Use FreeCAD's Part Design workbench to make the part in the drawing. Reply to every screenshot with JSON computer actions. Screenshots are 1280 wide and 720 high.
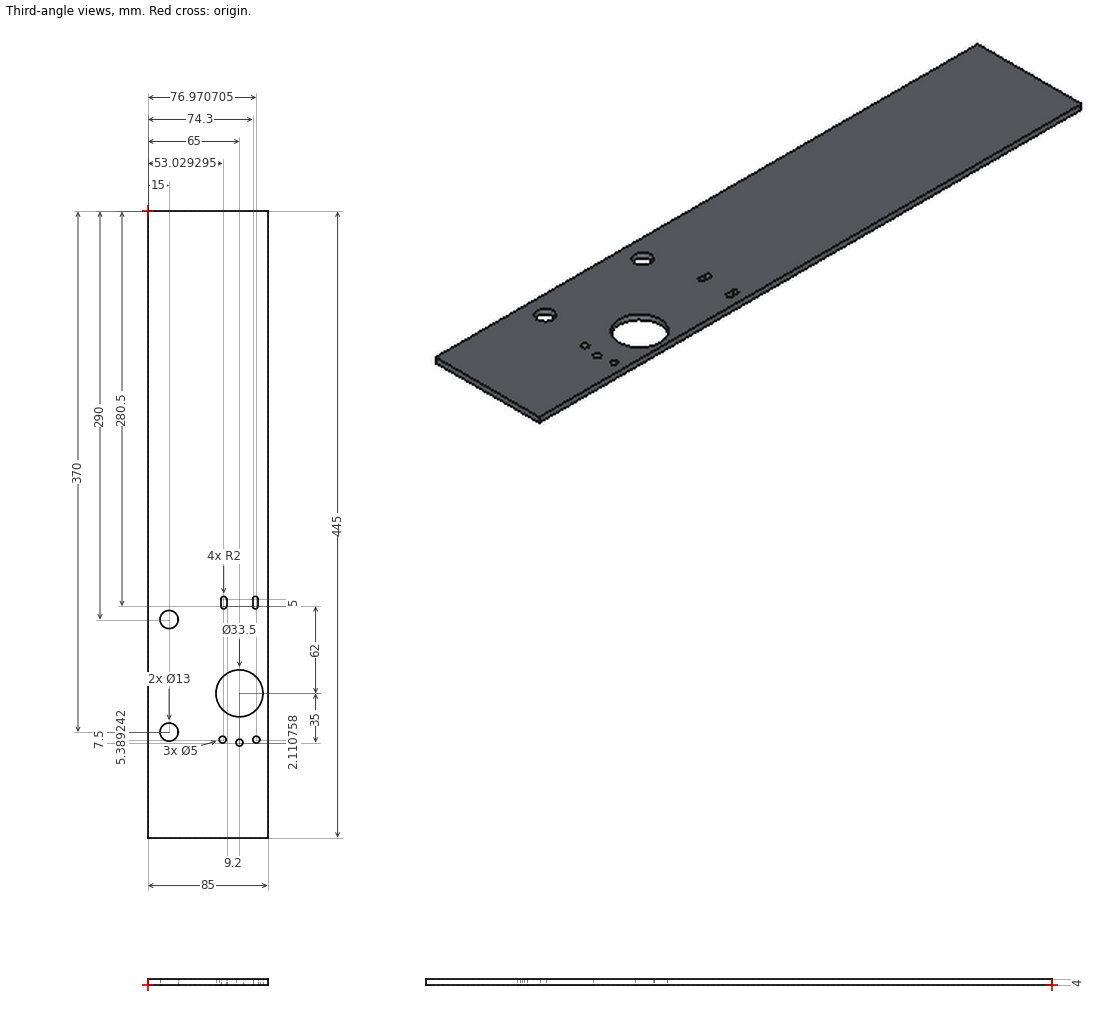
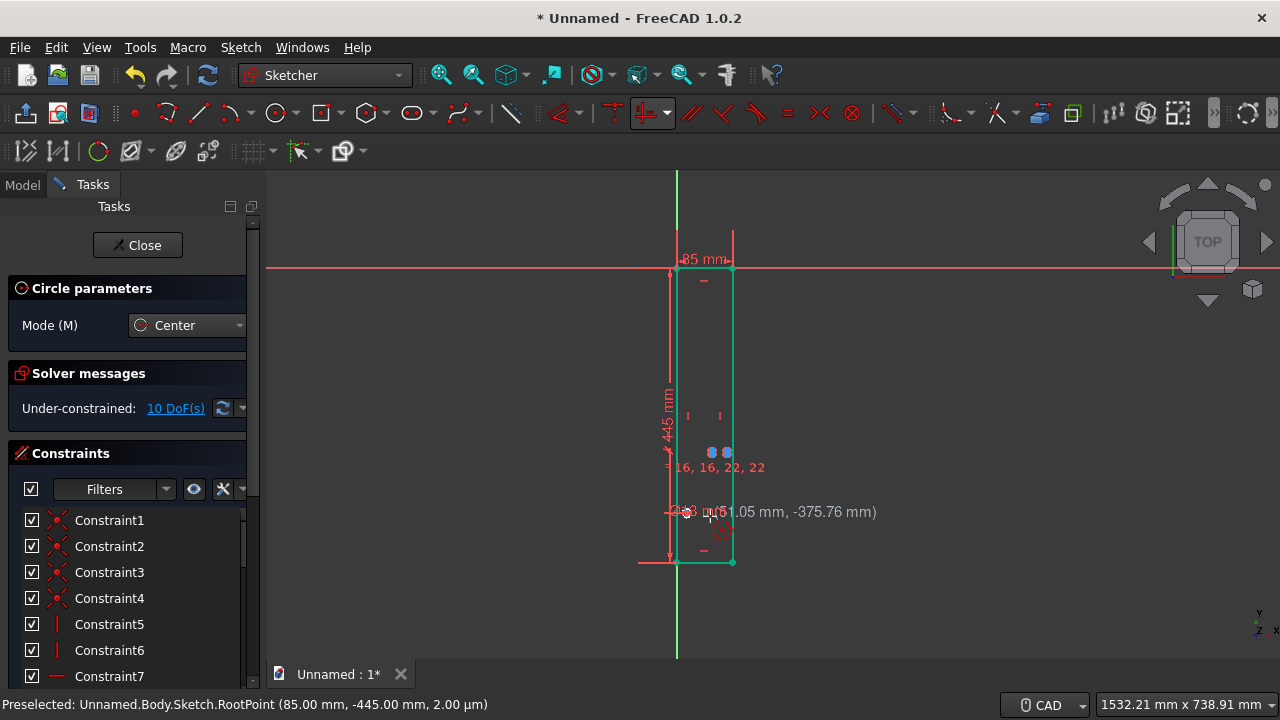
{"action": "left_click", "coordinate": [712, 516]}
{"action": "mouse_move", "coordinate": [713, 515]}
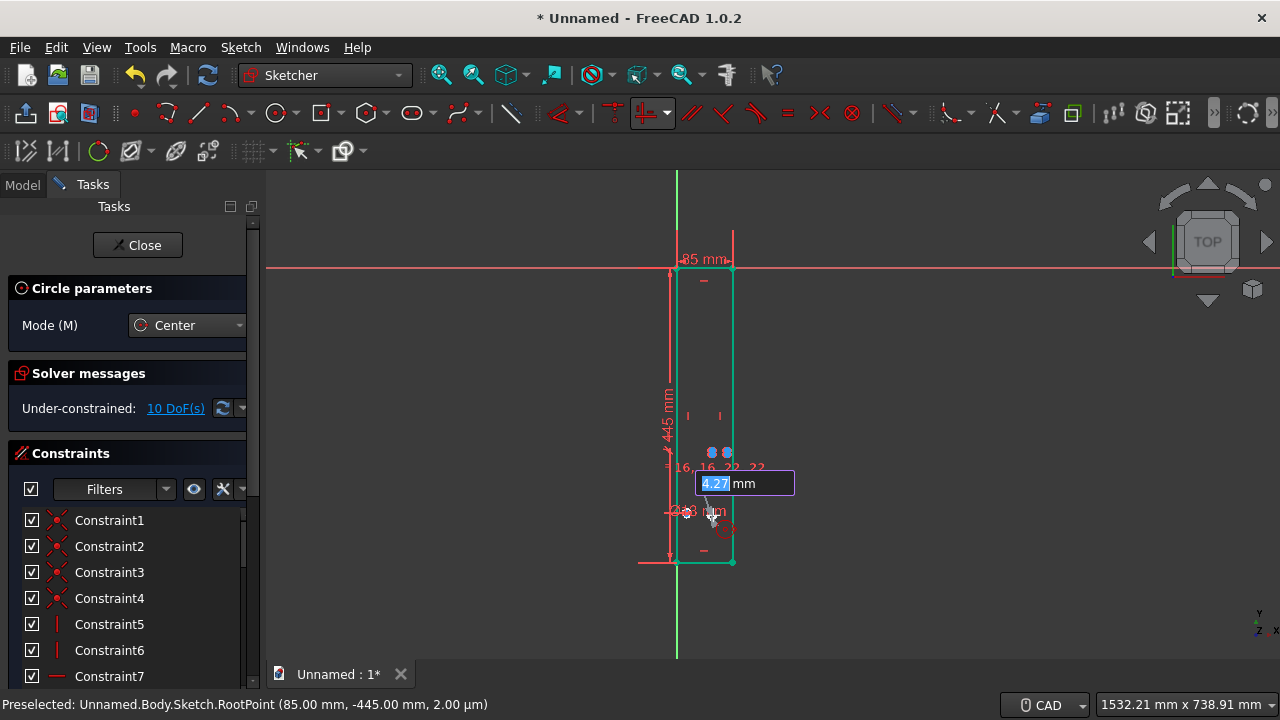
{"action": "type", "text": "5"}
{"action": "key", "text": "Return"}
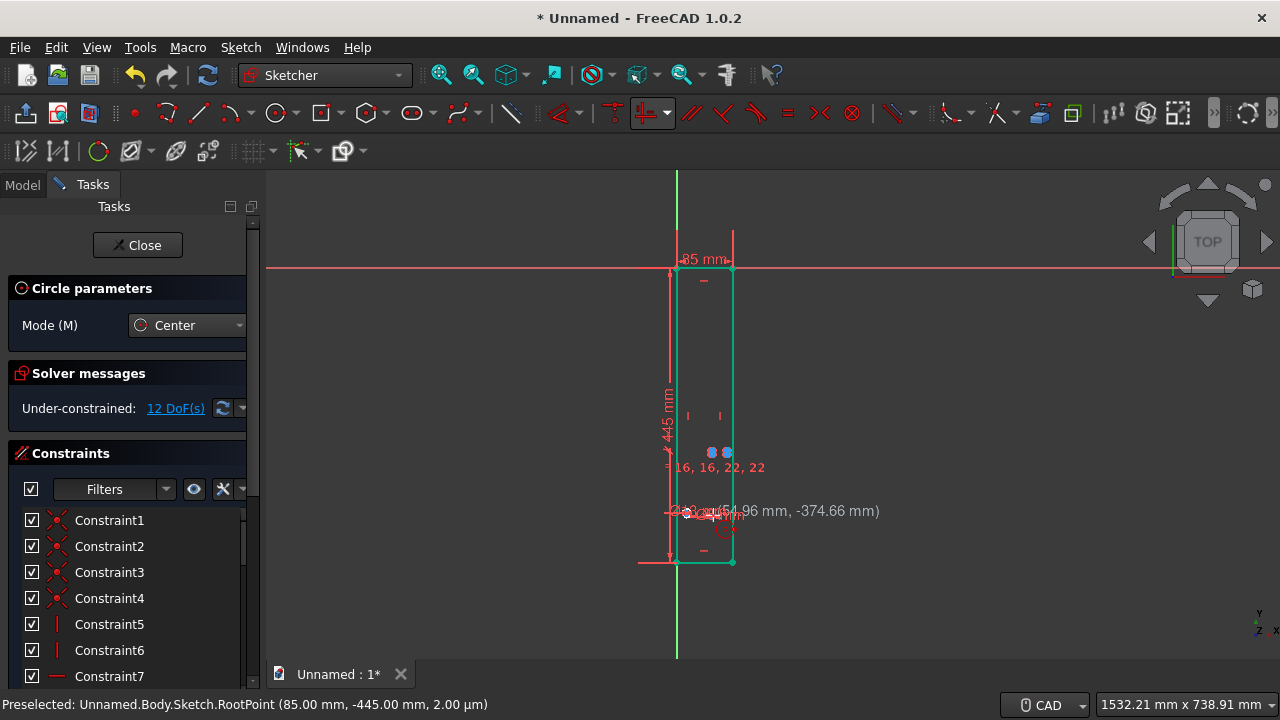
{"action": "scroll", "coordinate": [720, 518], "scroll_direction": "up", "scroll_amount": 14}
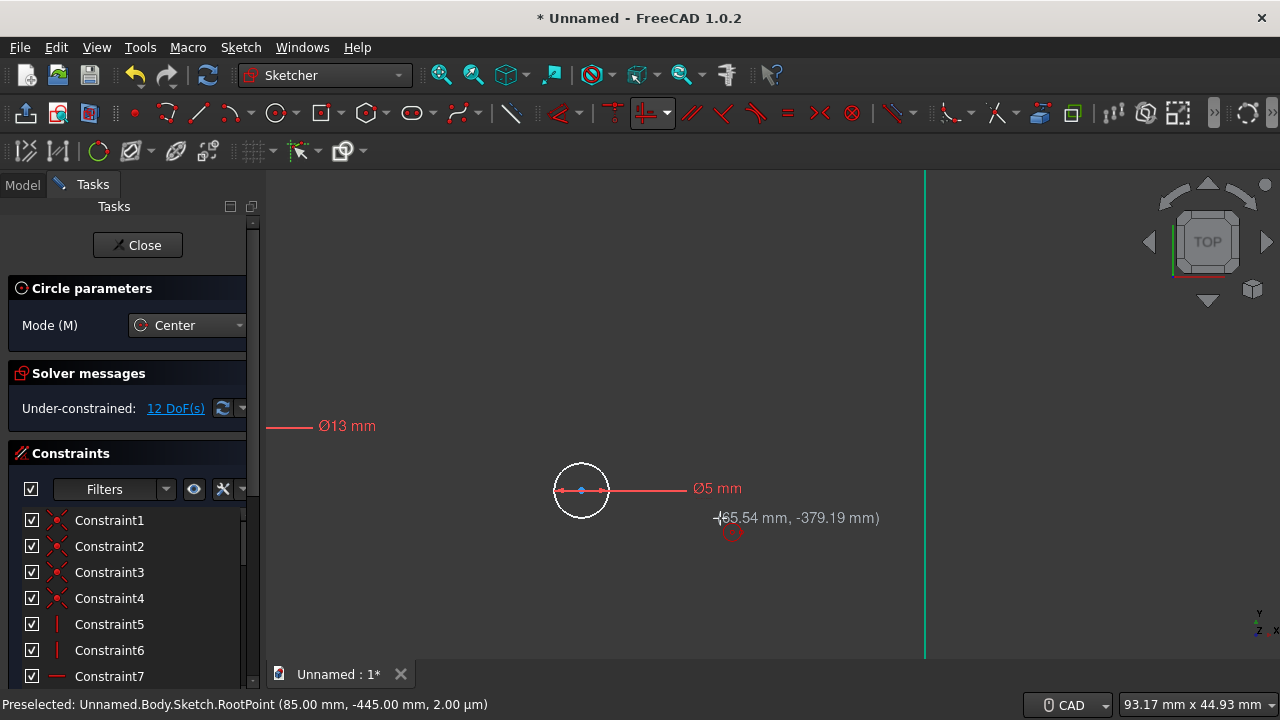
{"action": "scroll", "coordinate": [720, 518], "scroll_direction": "down", "scroll_amount": 14}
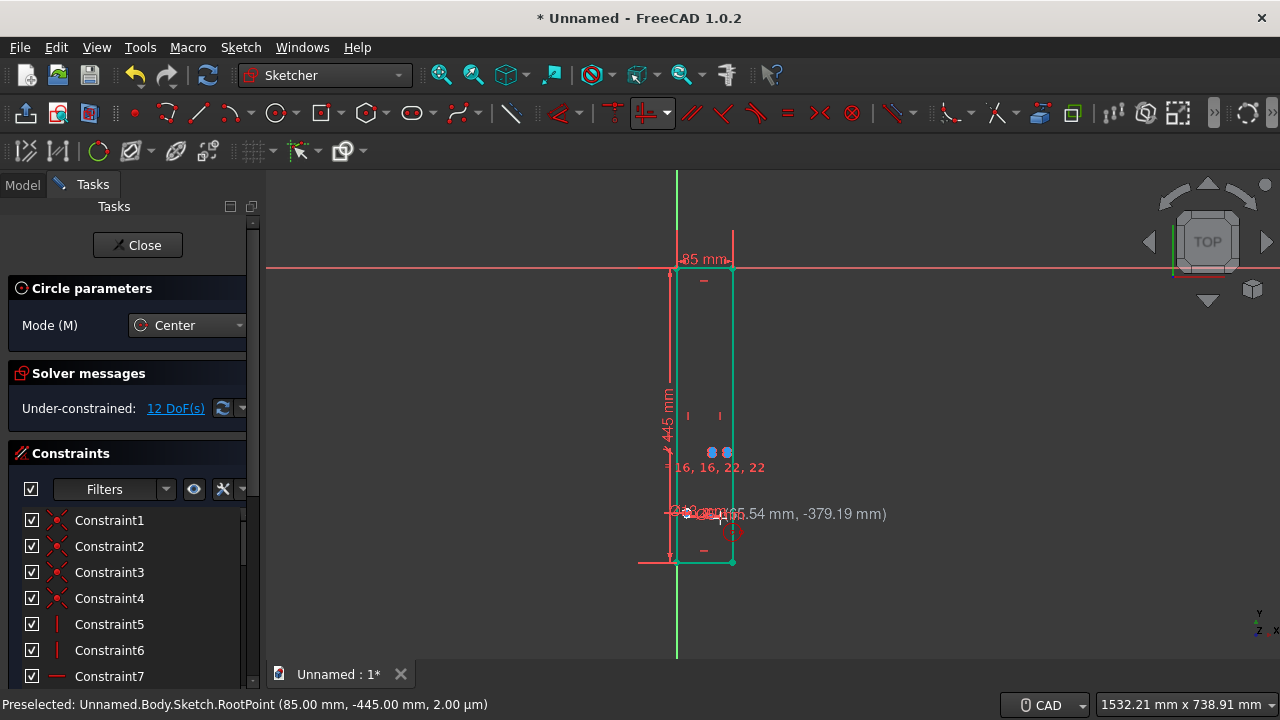
{"action": "scroll", "coordinate": [720, 518], "scroll_direction": "up", "scroll_amount": 5}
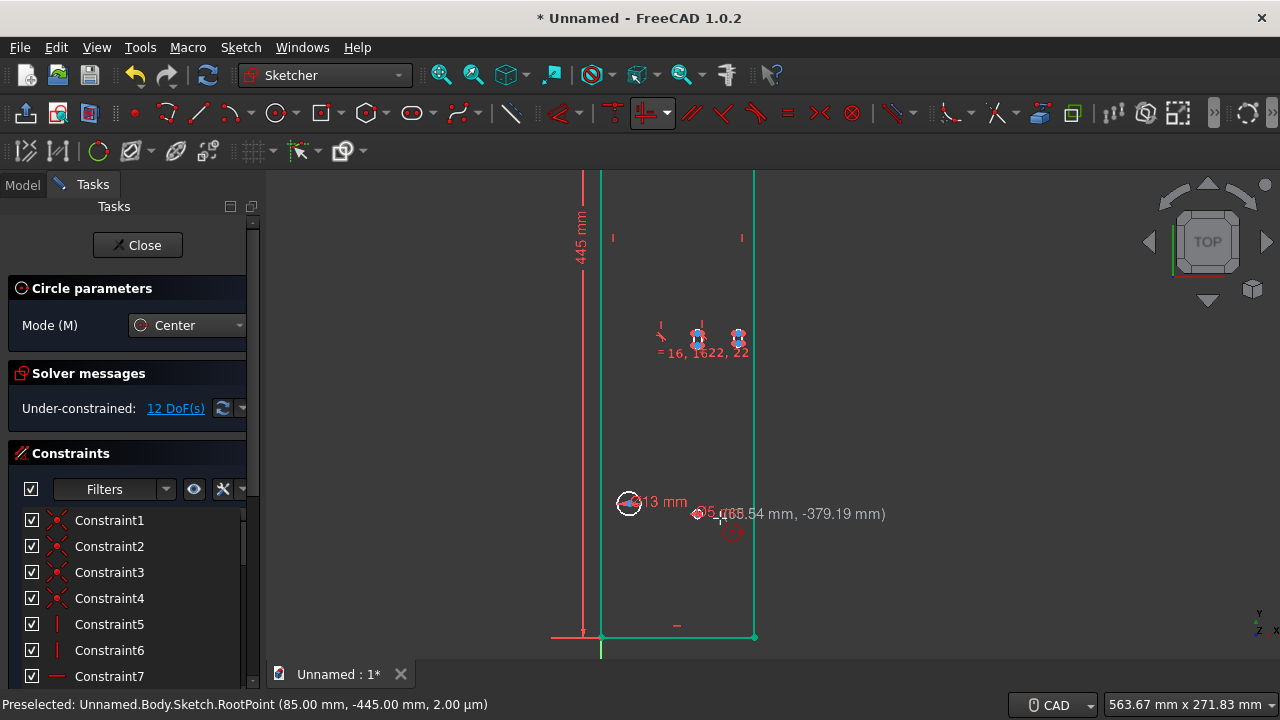
{"action": "left_click", "coordinate": [718, 516]}
{"action": "mouse_move", "coordinate": [721, 513]}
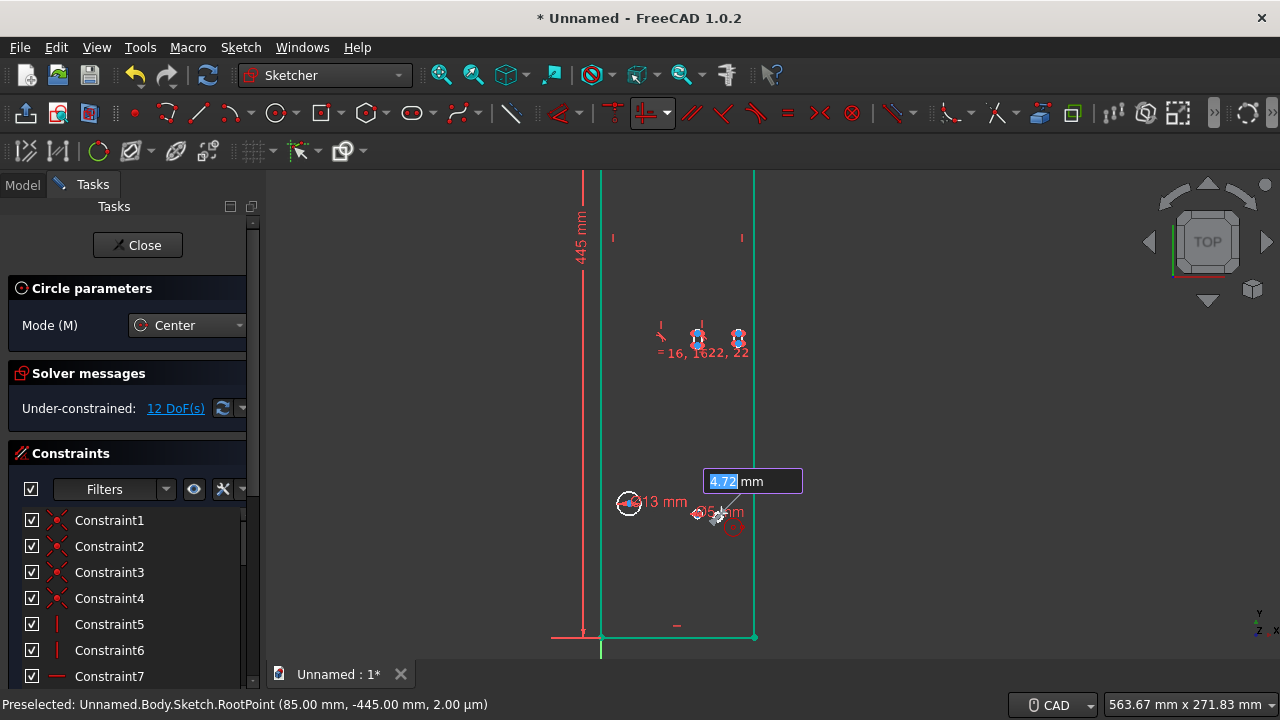
{"action": "type", "text": "5"}
{"action": "key", "text": "Return"}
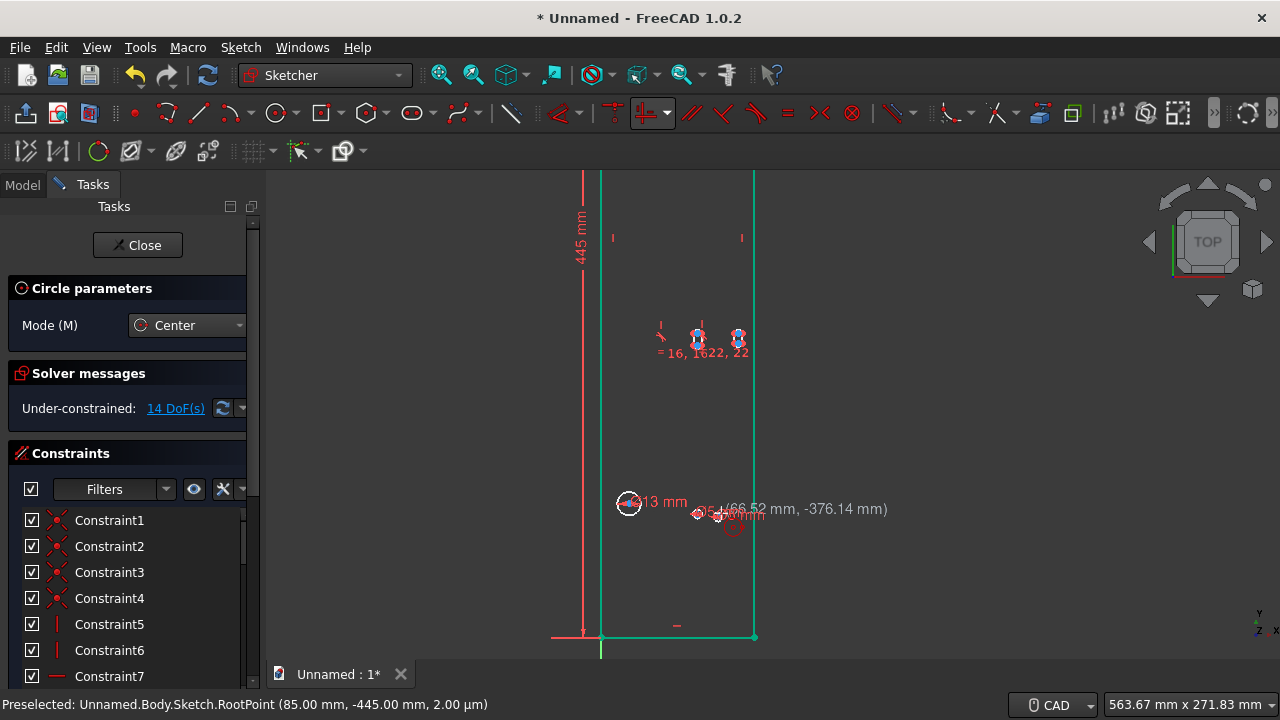
{"action": "scroll", "coordinate": [740, 513], "scroll_direction": "up", "scroll_amount": 9}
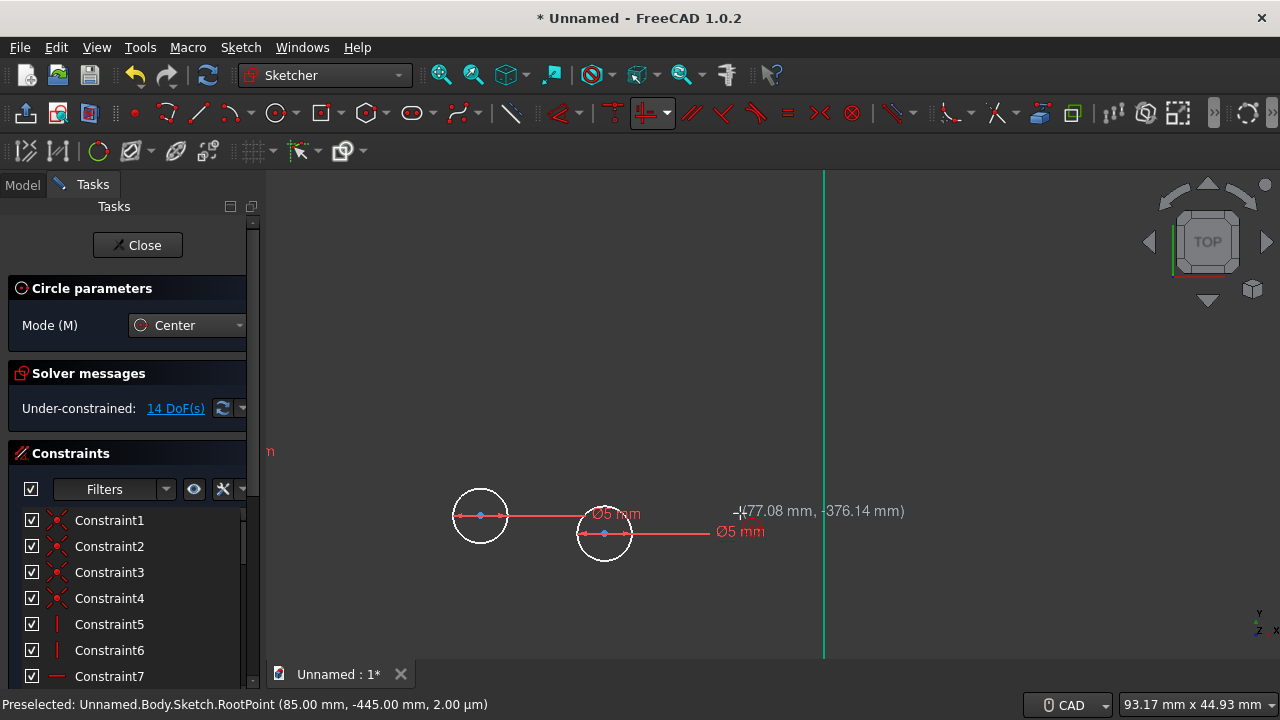
{"action": "scroll", "coordinate": [727, 516], "scroll_direction": "down", "scroll_amount": 14}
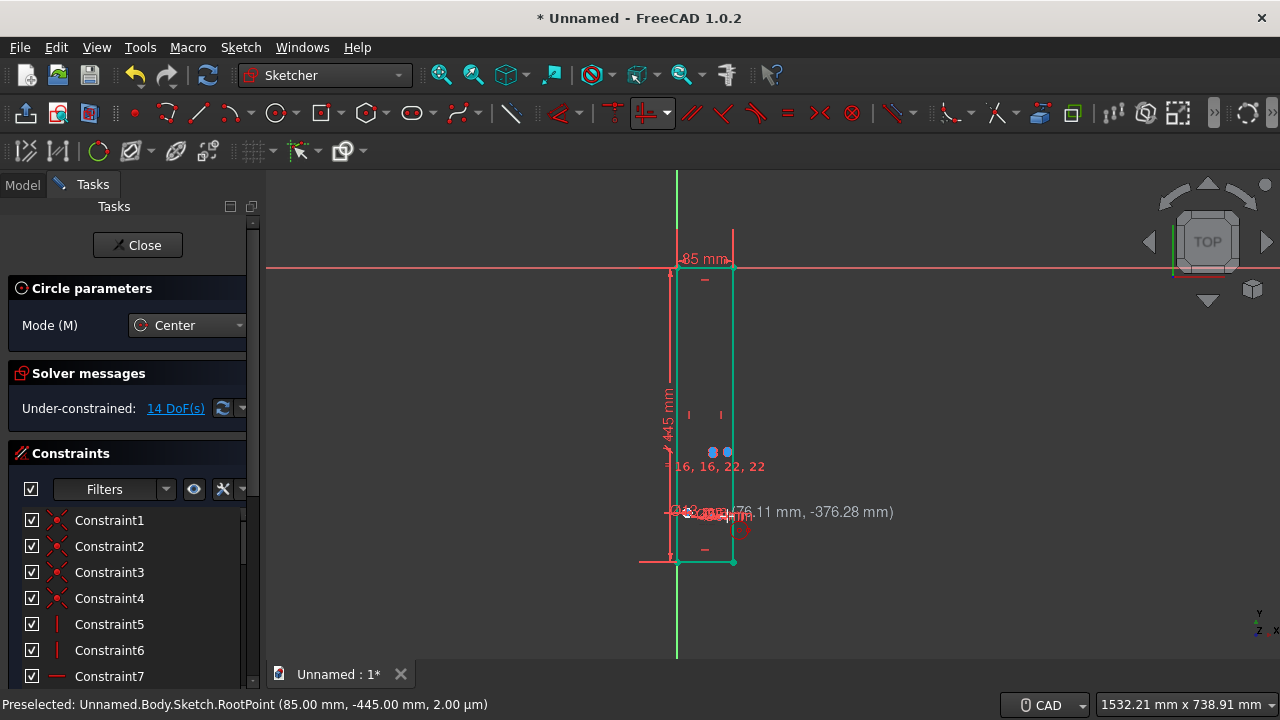
{"action": "scroll", "coordinate": [728, 516], "scroll_direction": "up", "scroll_amount": 6}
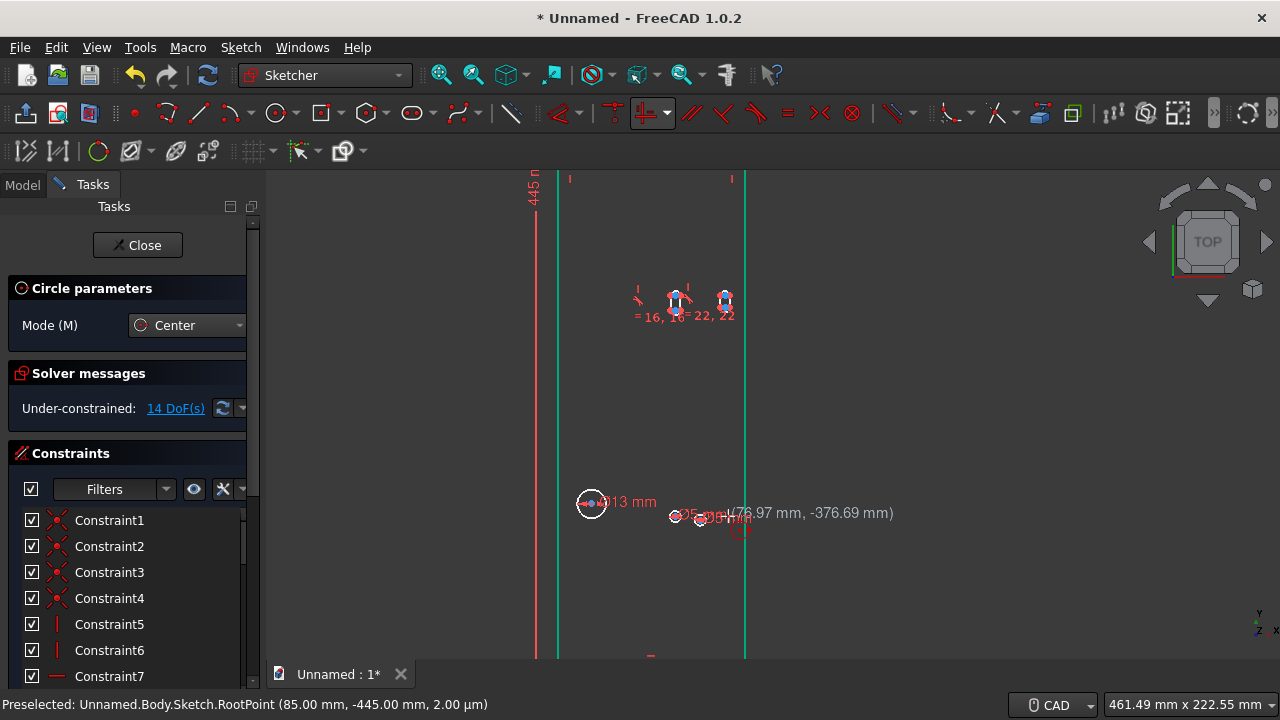
{"action": "left_click", "coordinate": [727, 515]}
{"action": "mouse_move", "coordinate": [723, 511]}